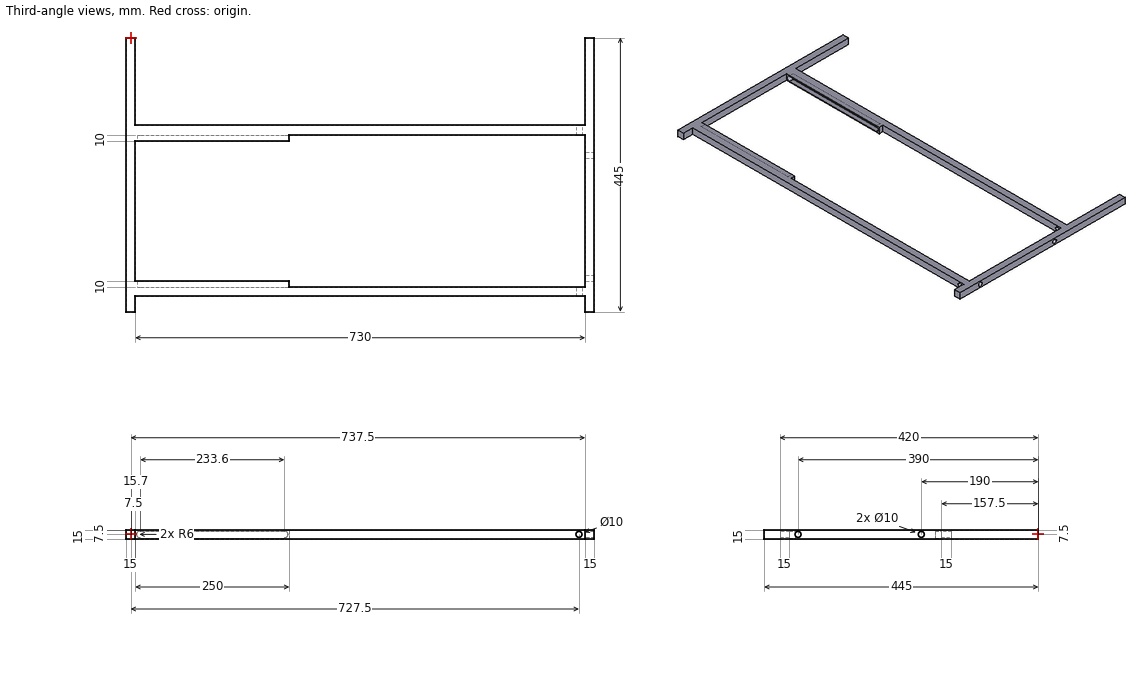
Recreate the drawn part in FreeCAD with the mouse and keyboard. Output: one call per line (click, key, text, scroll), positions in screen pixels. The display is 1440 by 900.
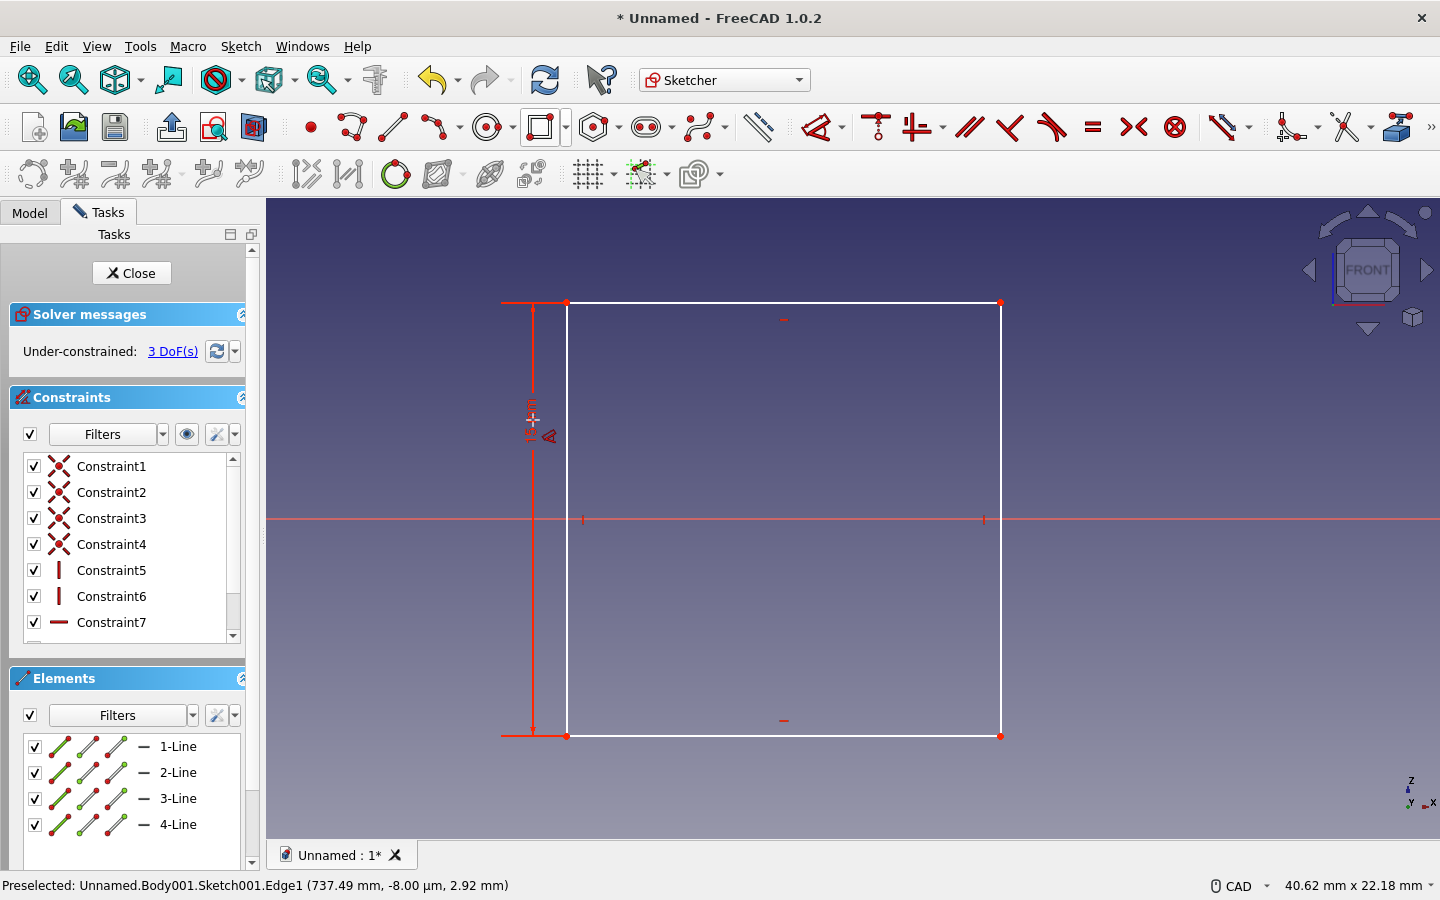
click(697, 736)
click(784, 770)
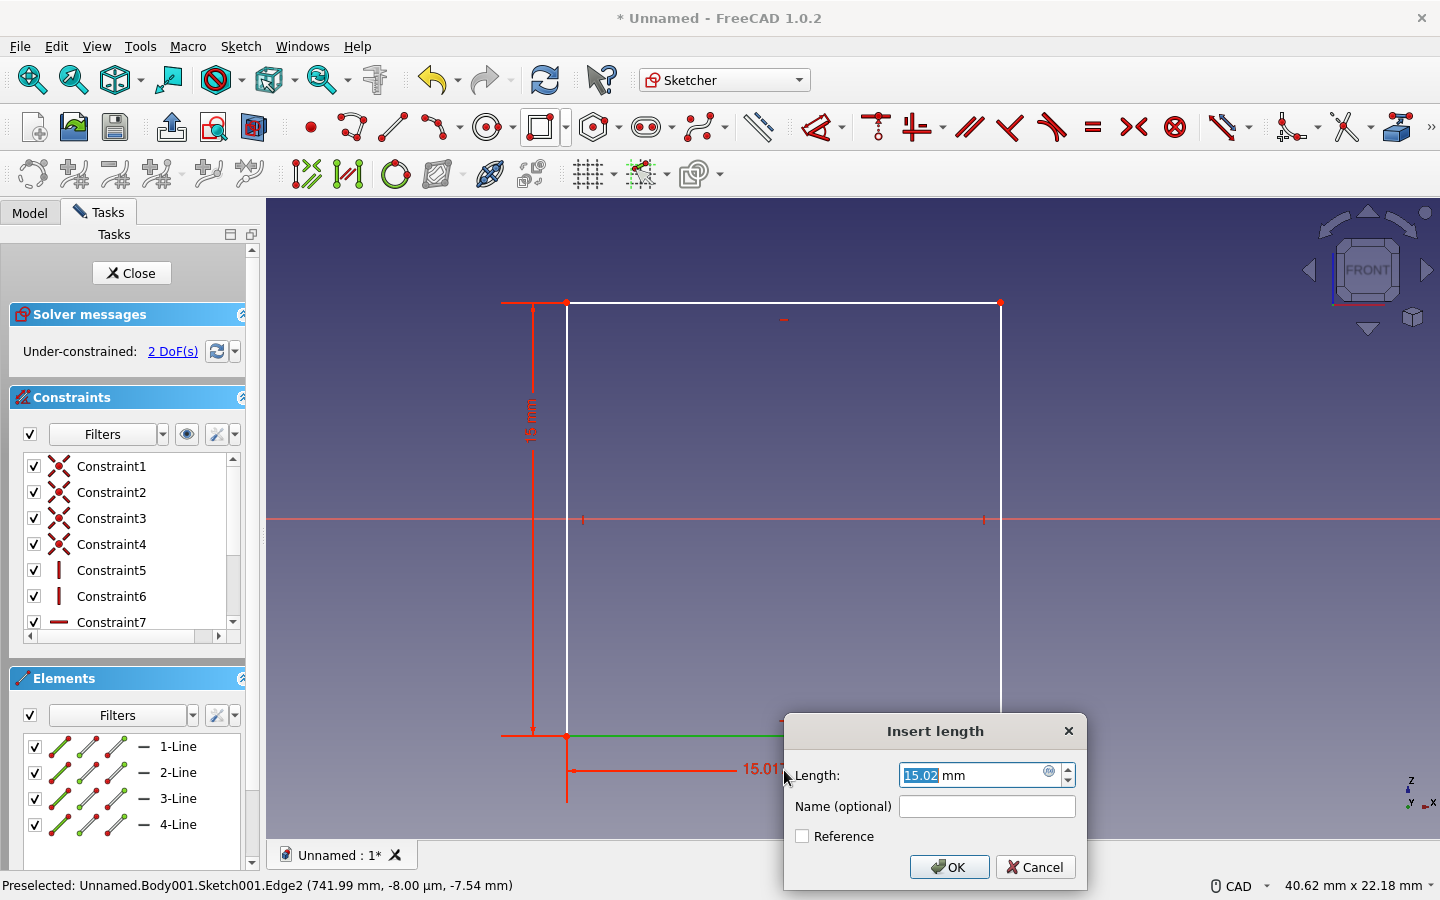
text(15)
key(Return)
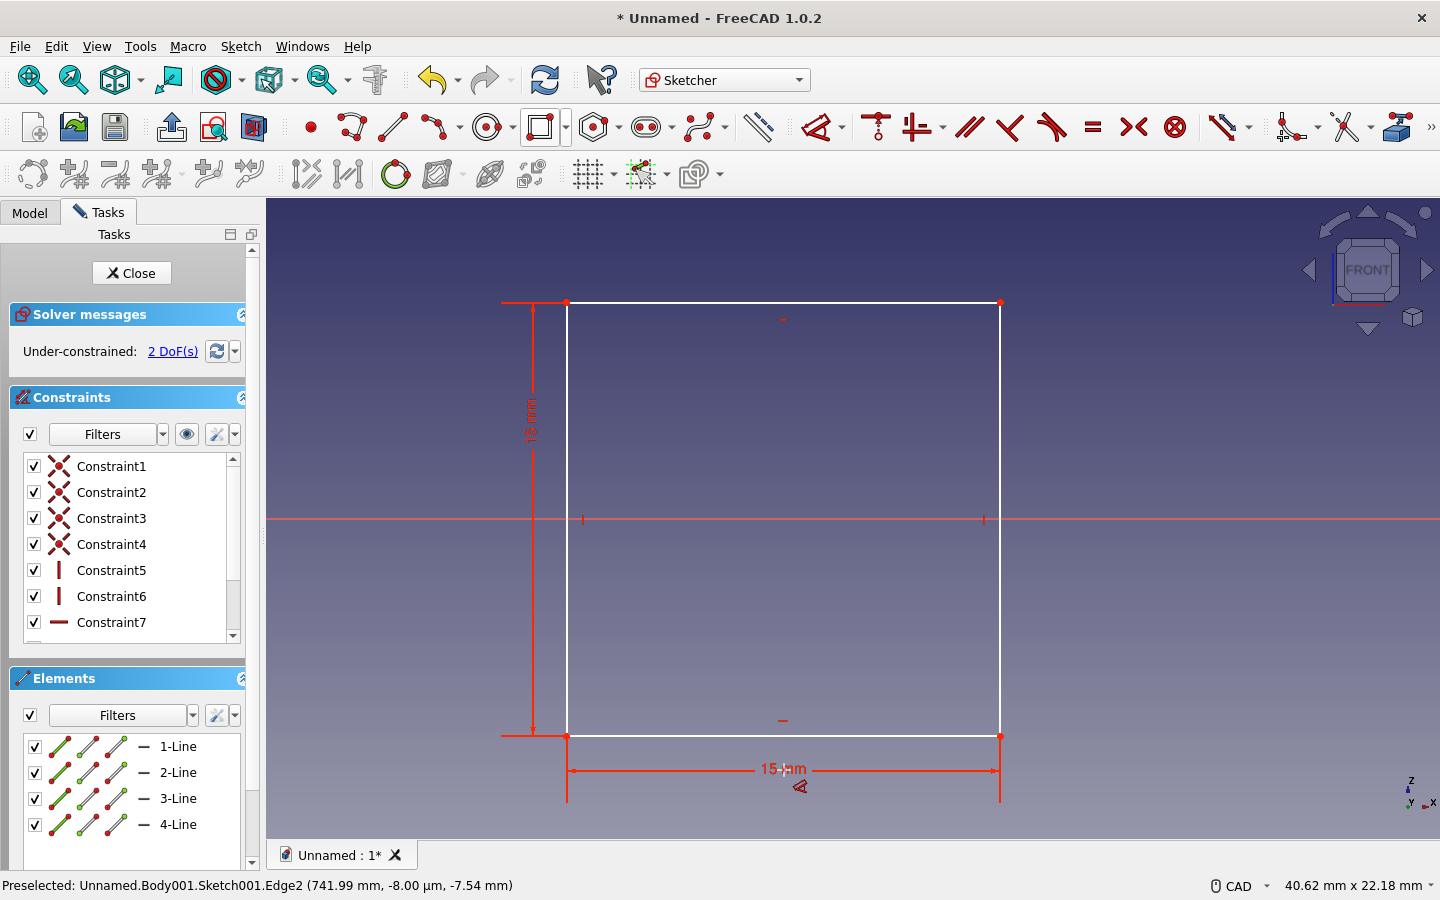
click(567, 303)
click(601, 361)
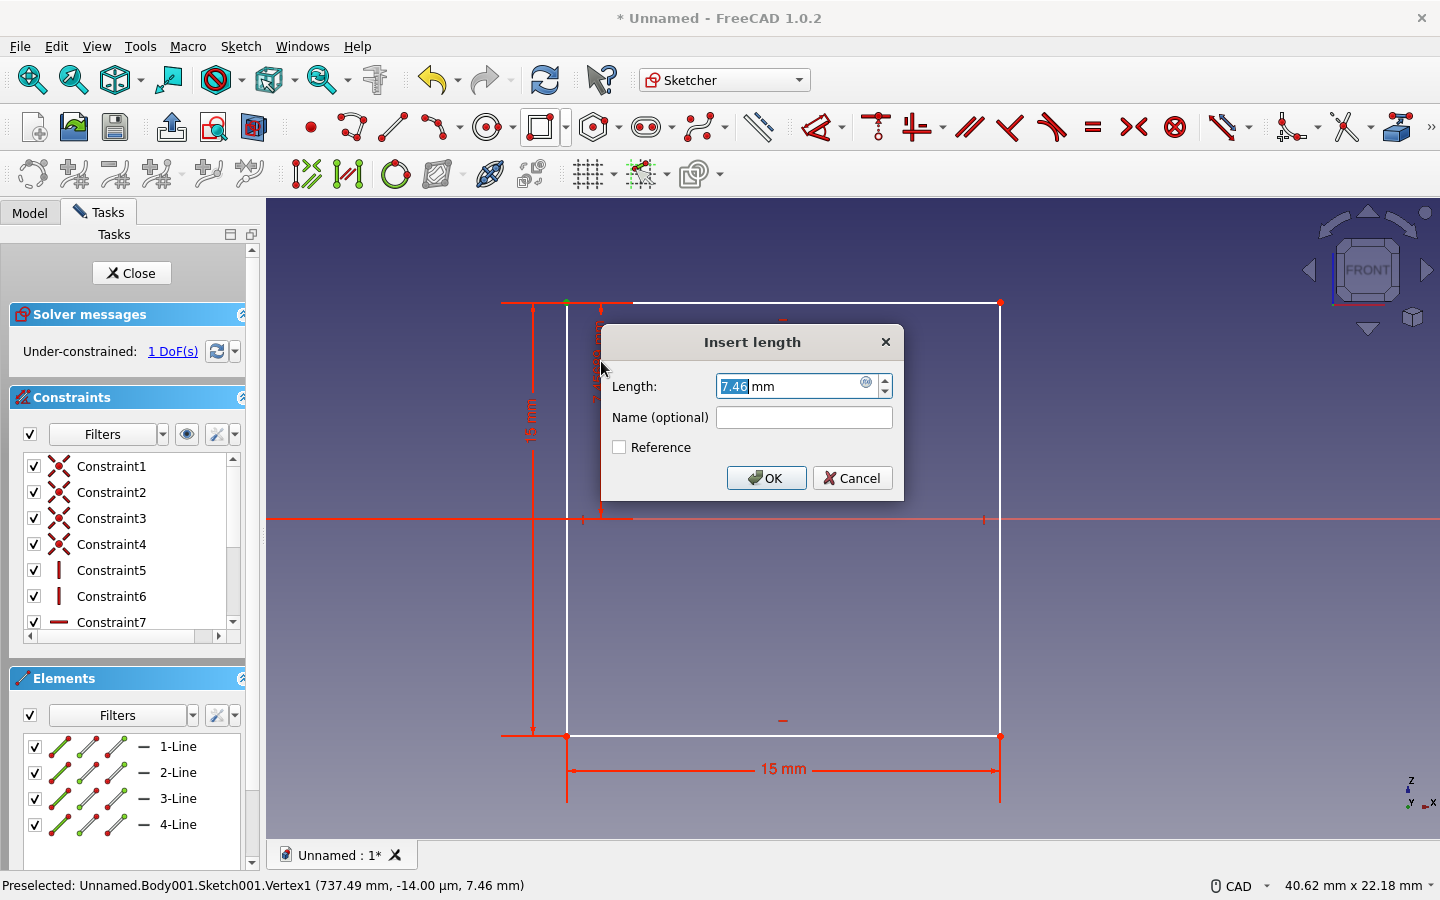
text(7.5)
key(Return)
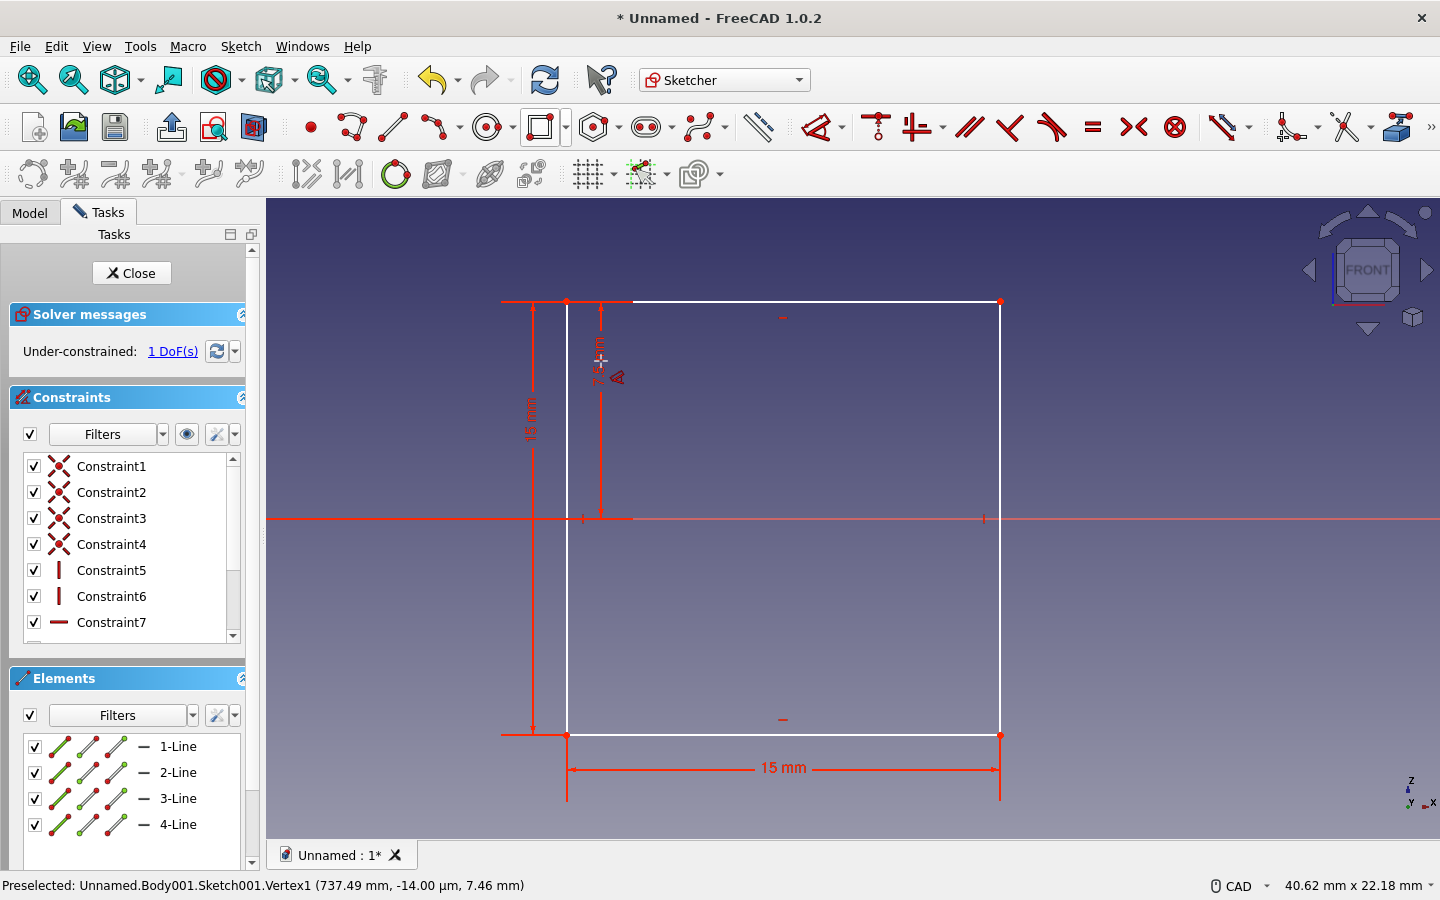
click(567, 302)
click(430, 268)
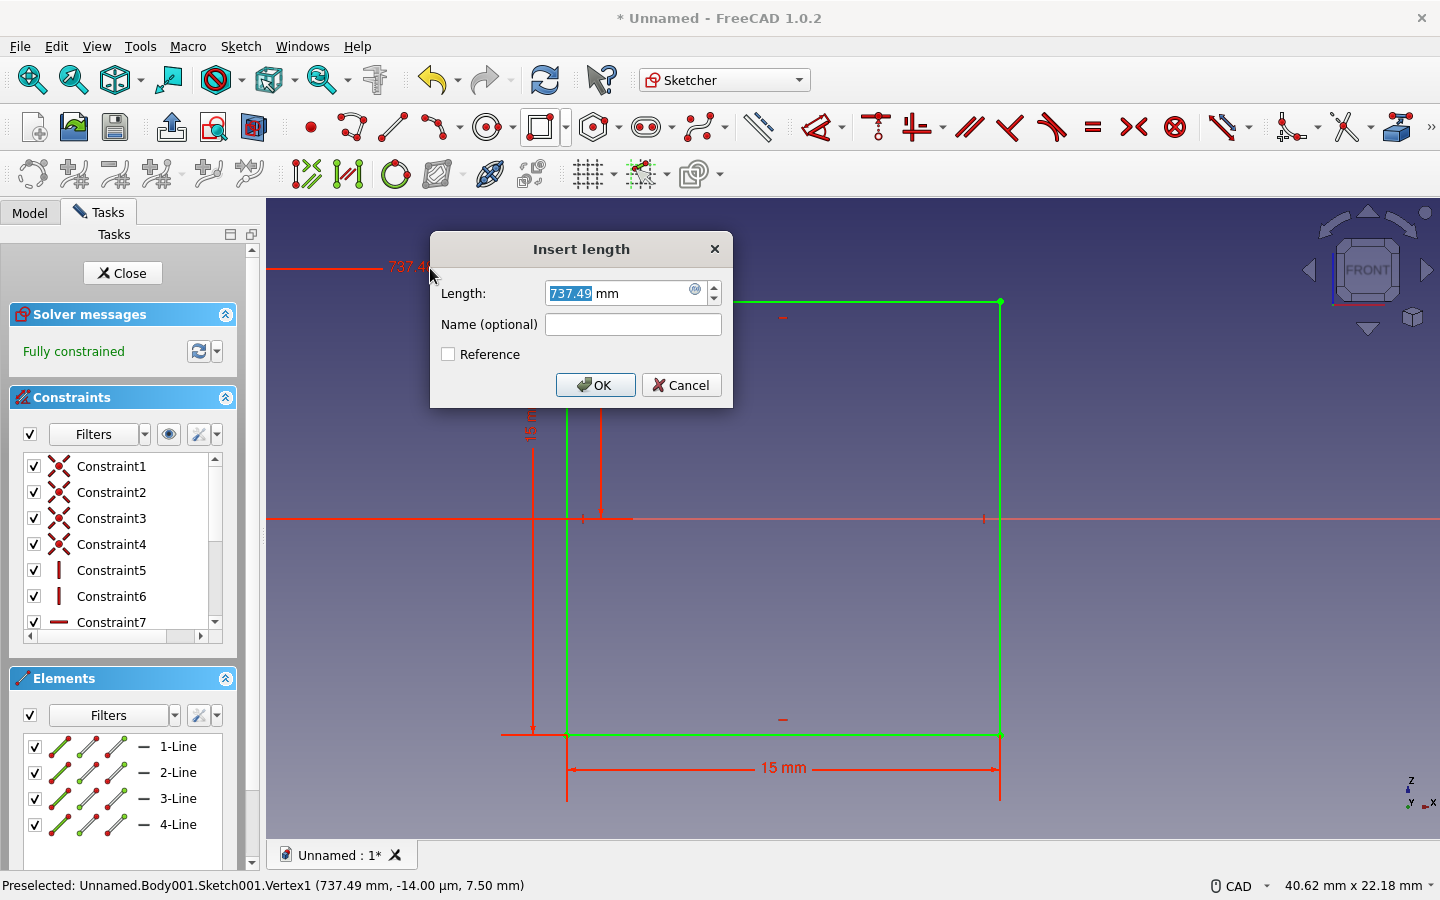
text(737.5)
key(Return)
key(Escape)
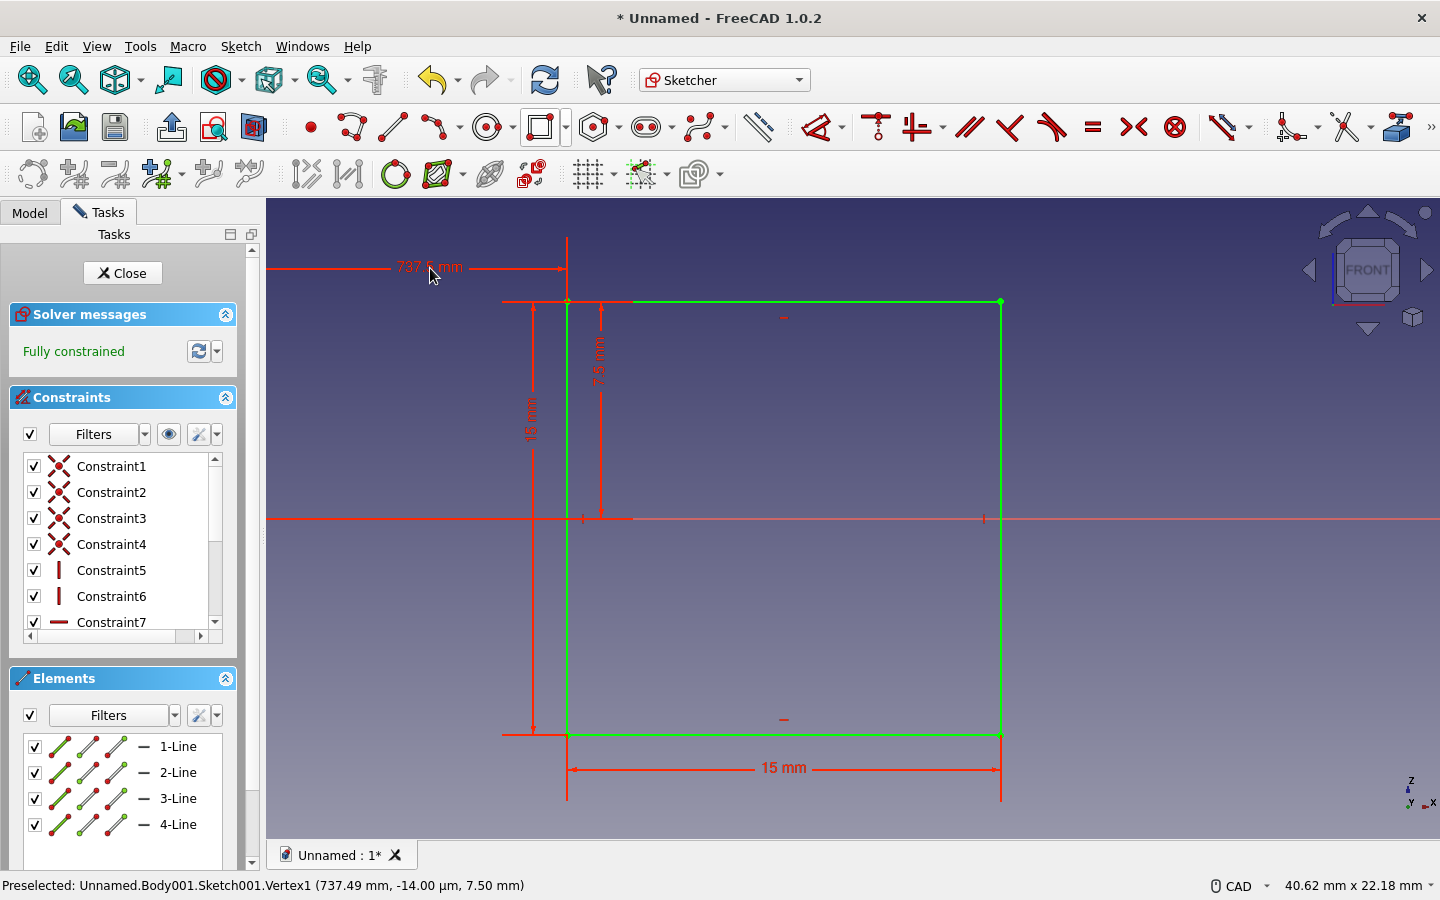
click(123, 273)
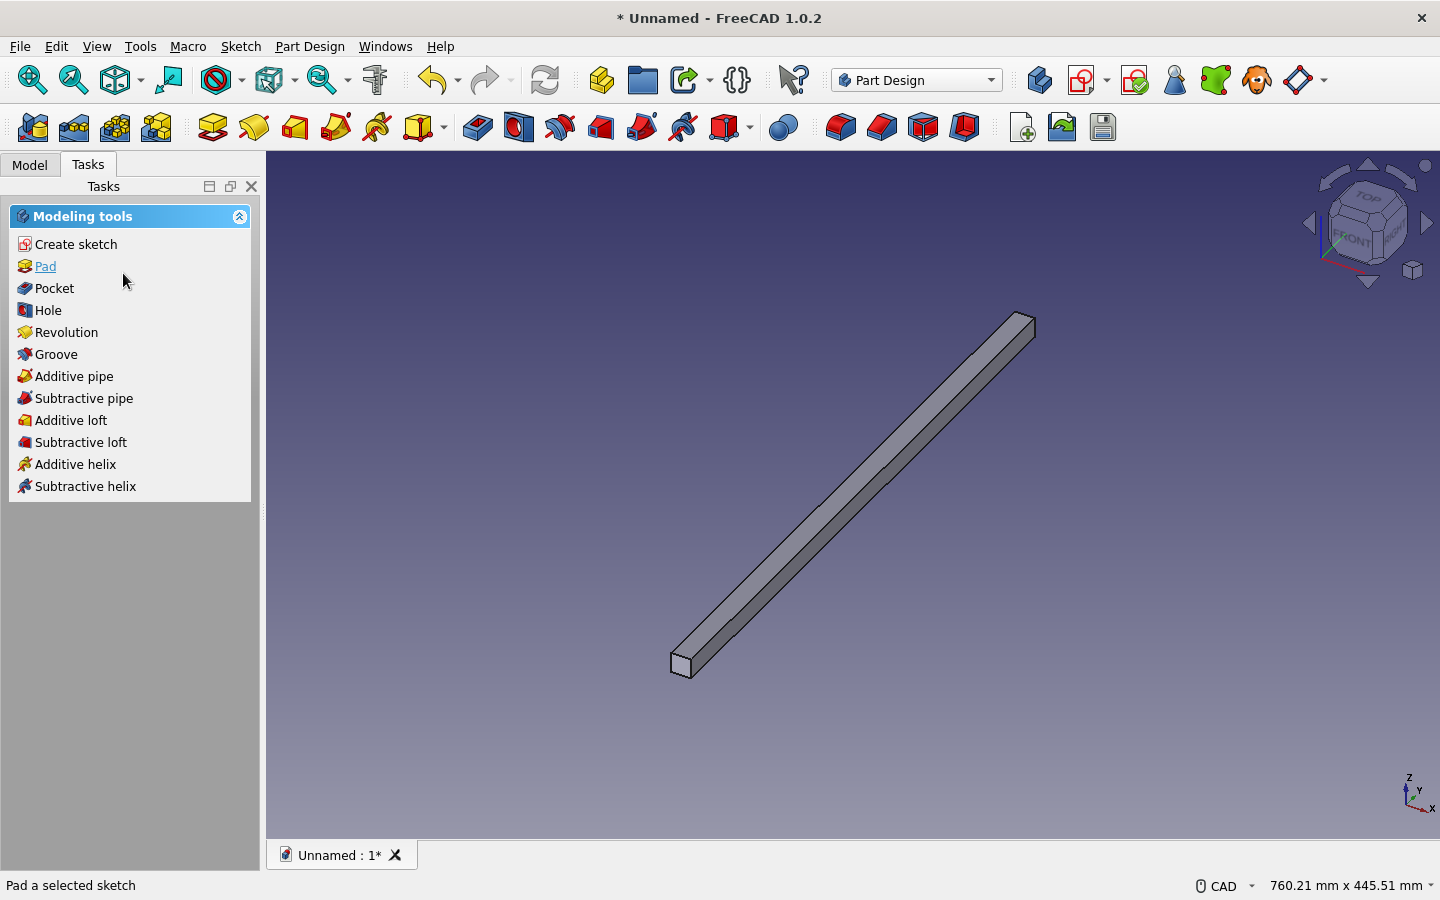
click(213, 128)